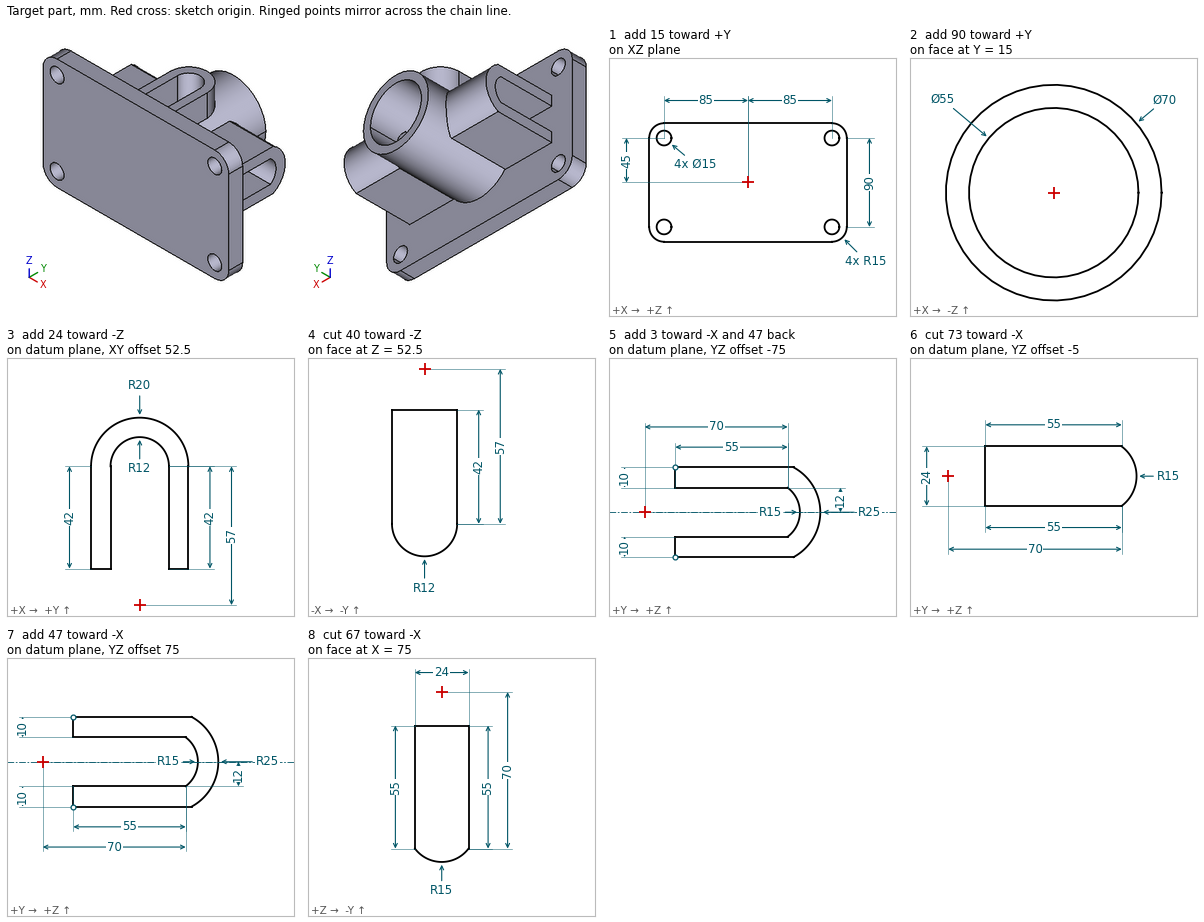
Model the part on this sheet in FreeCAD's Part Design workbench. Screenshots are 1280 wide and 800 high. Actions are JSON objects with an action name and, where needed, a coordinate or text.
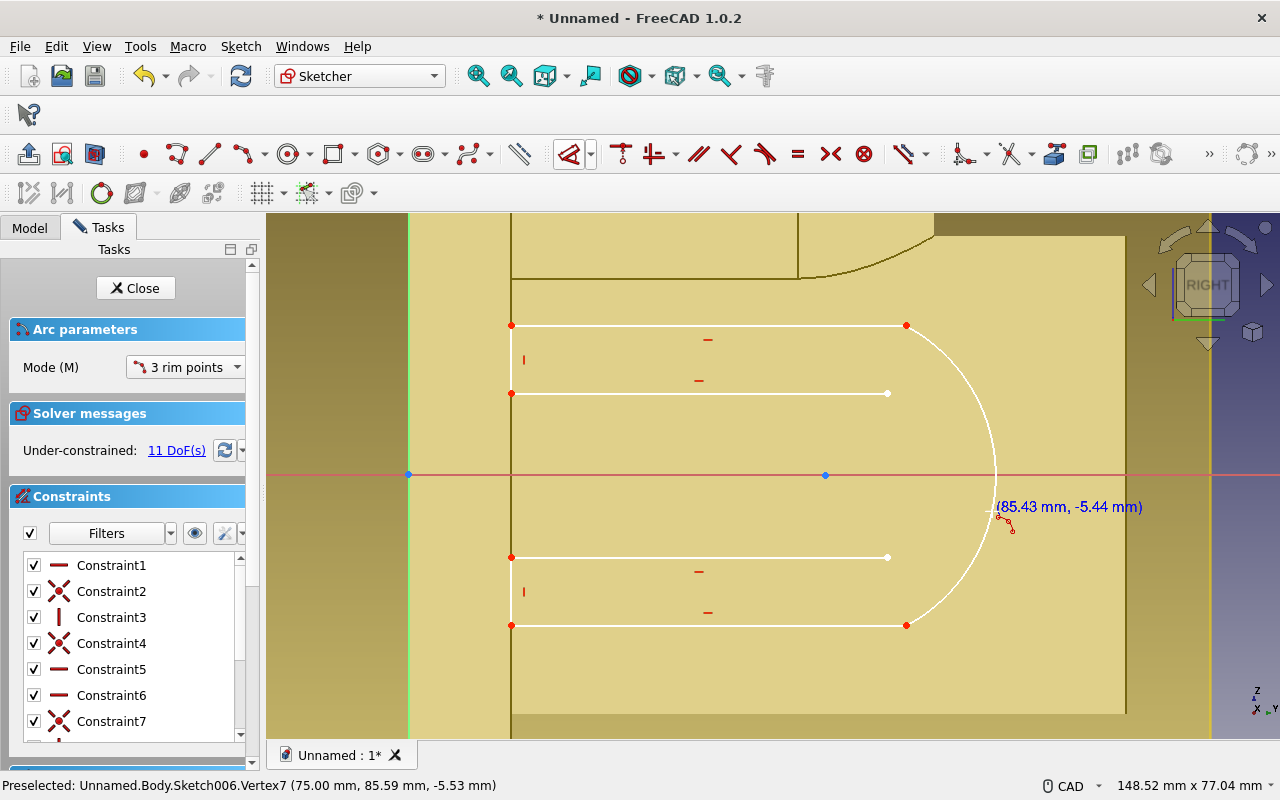
{"action": "left_click", "coordinate": [887, 394]}
{"action": "left_click", "coordinate": [887, 558]}
{"action": "left_click", "coordinate": [926, 494]}
{"action": "key", "text": "Escape"}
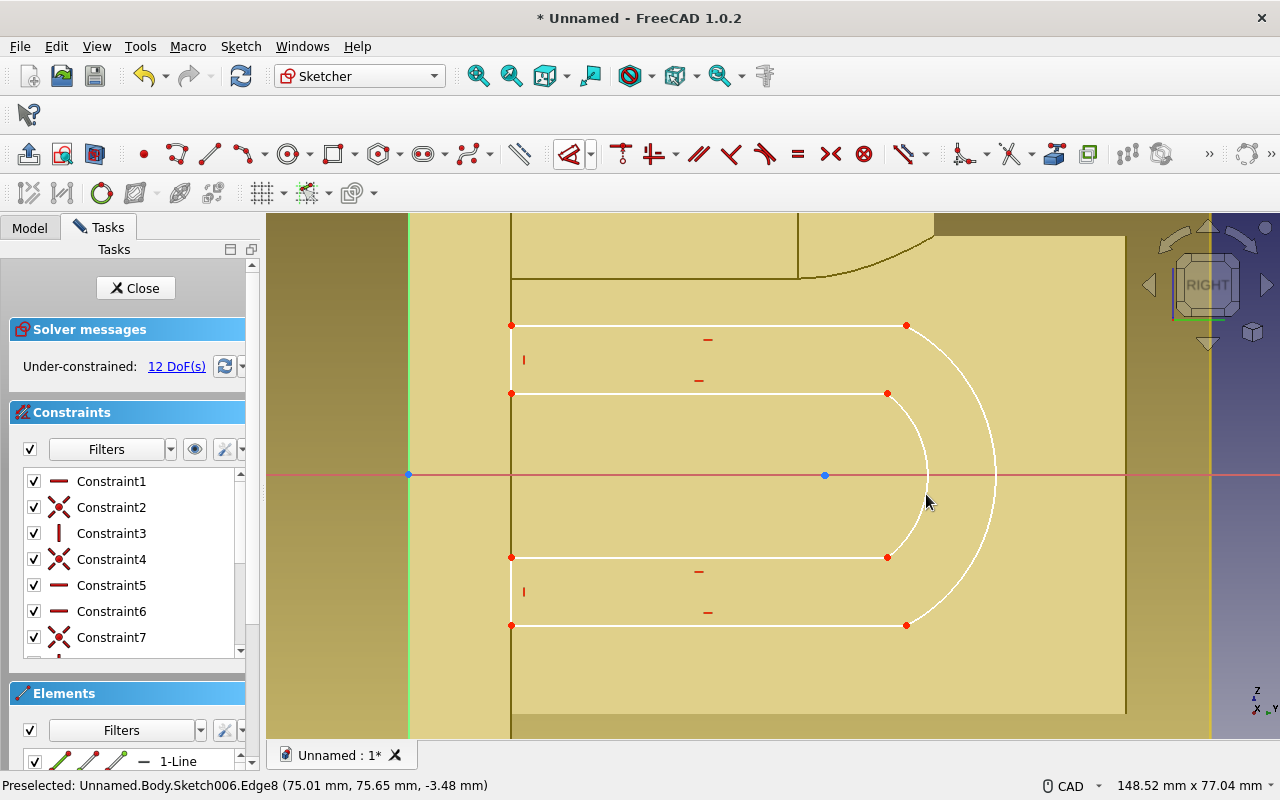
{"action": "left_click", "coordinate": [980, 547]}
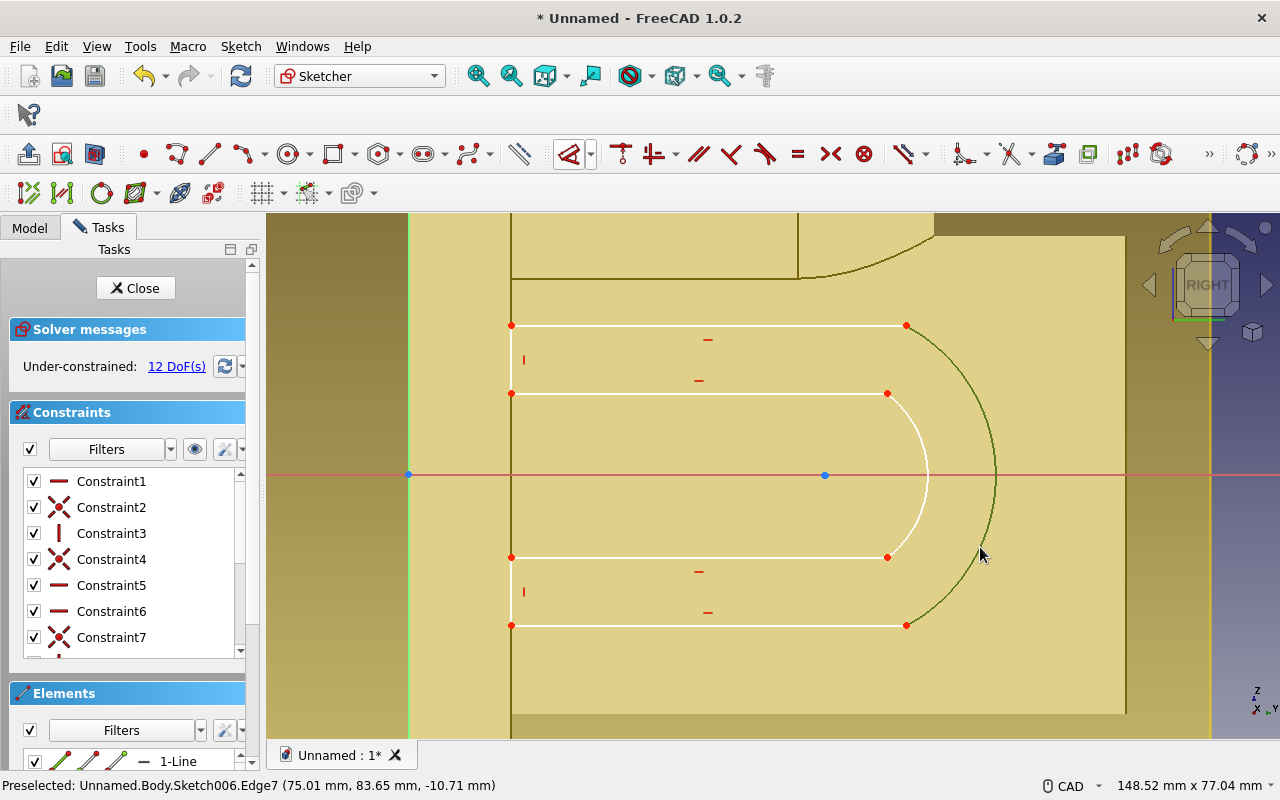
{"action": "left_click", "coordinate": [921, 513]}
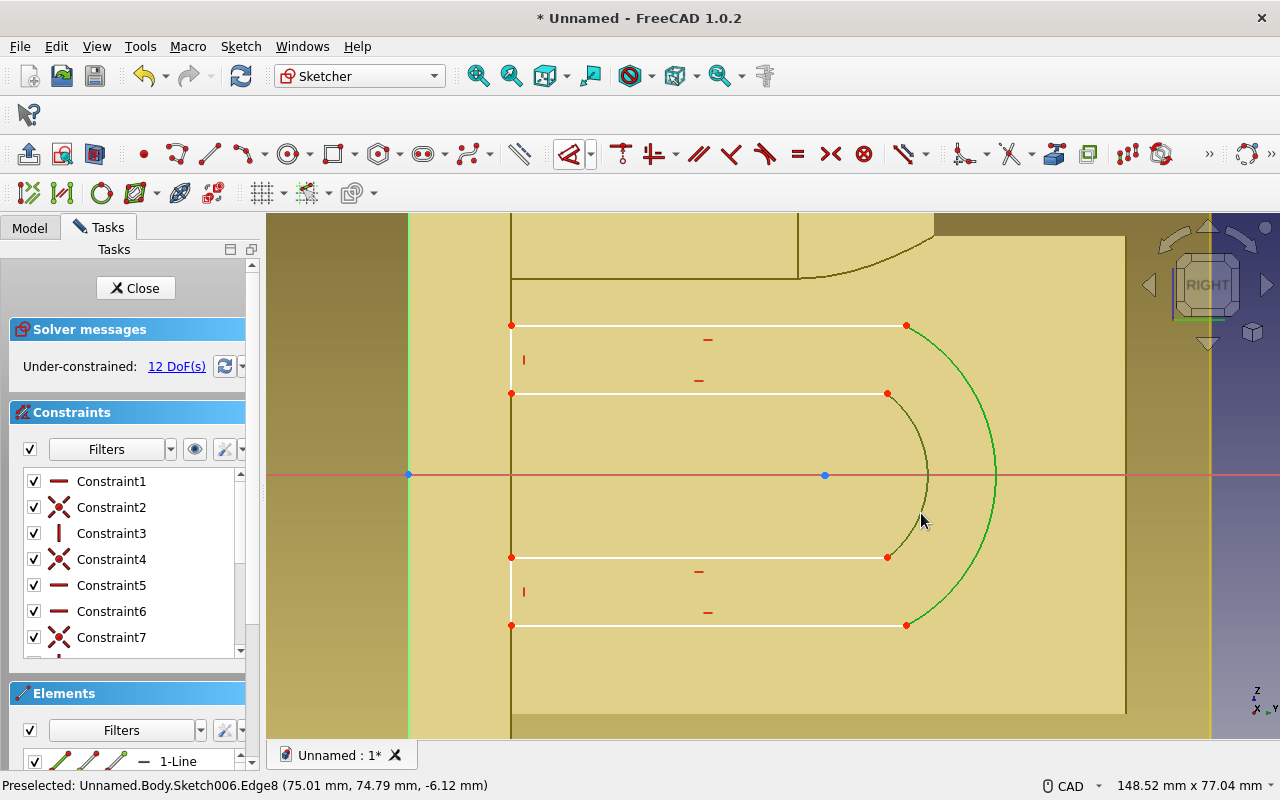
{"action": "key", "text": "c"}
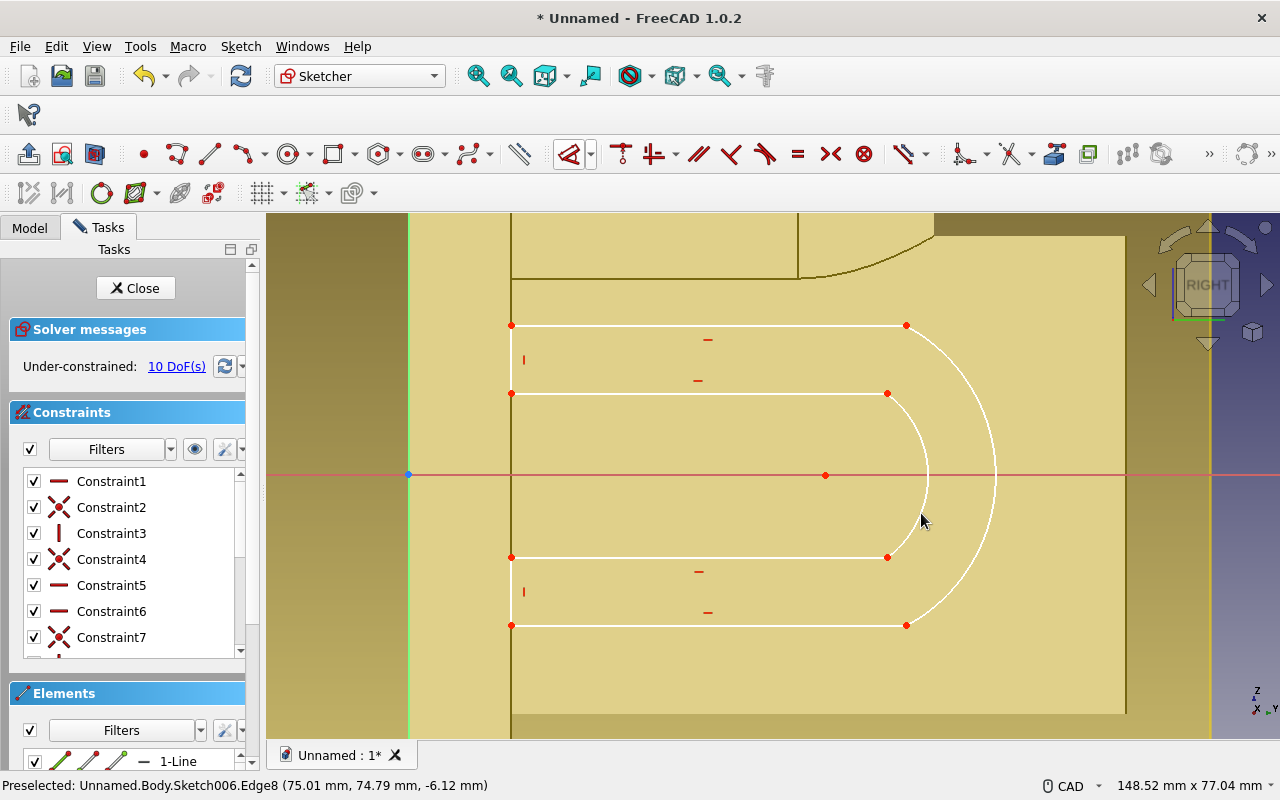
{"action": "left_click", "coordinate": [826, 476]}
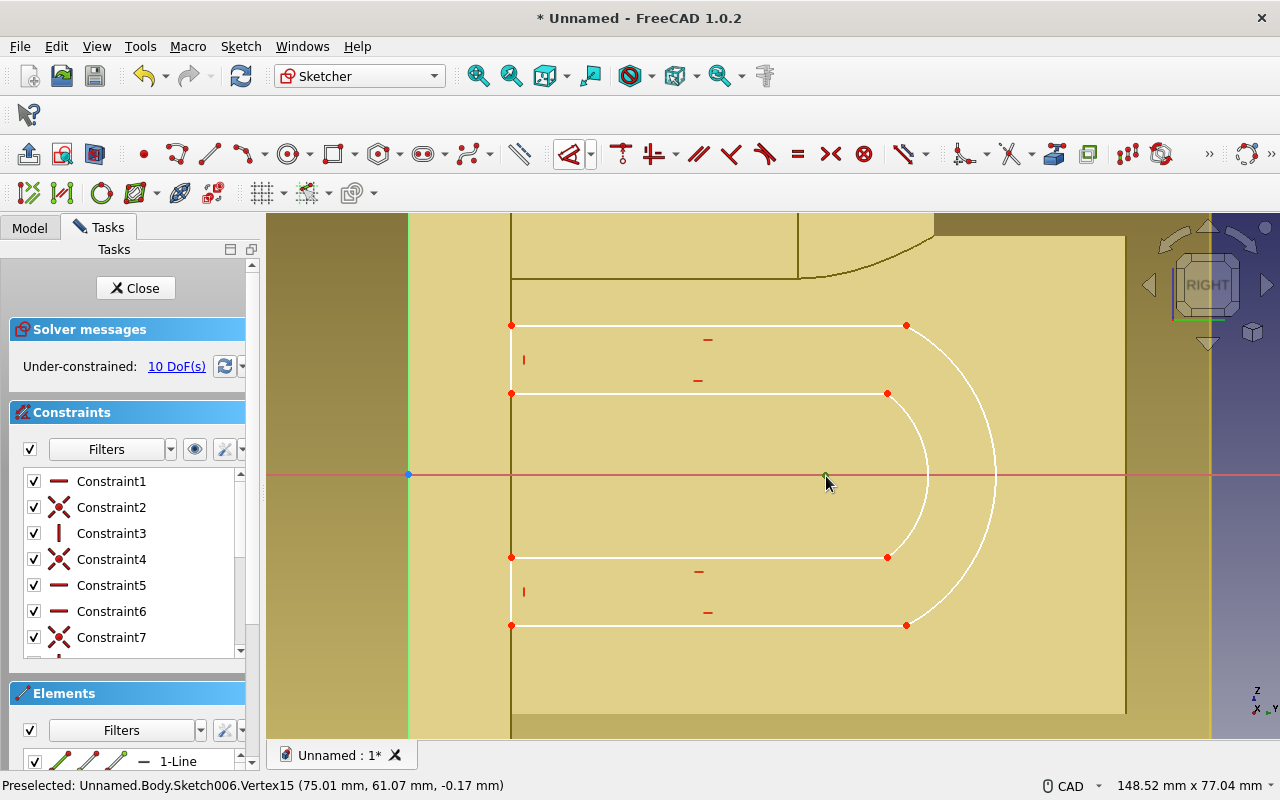
{"action": "left_click", "coordinate": [353, 475]}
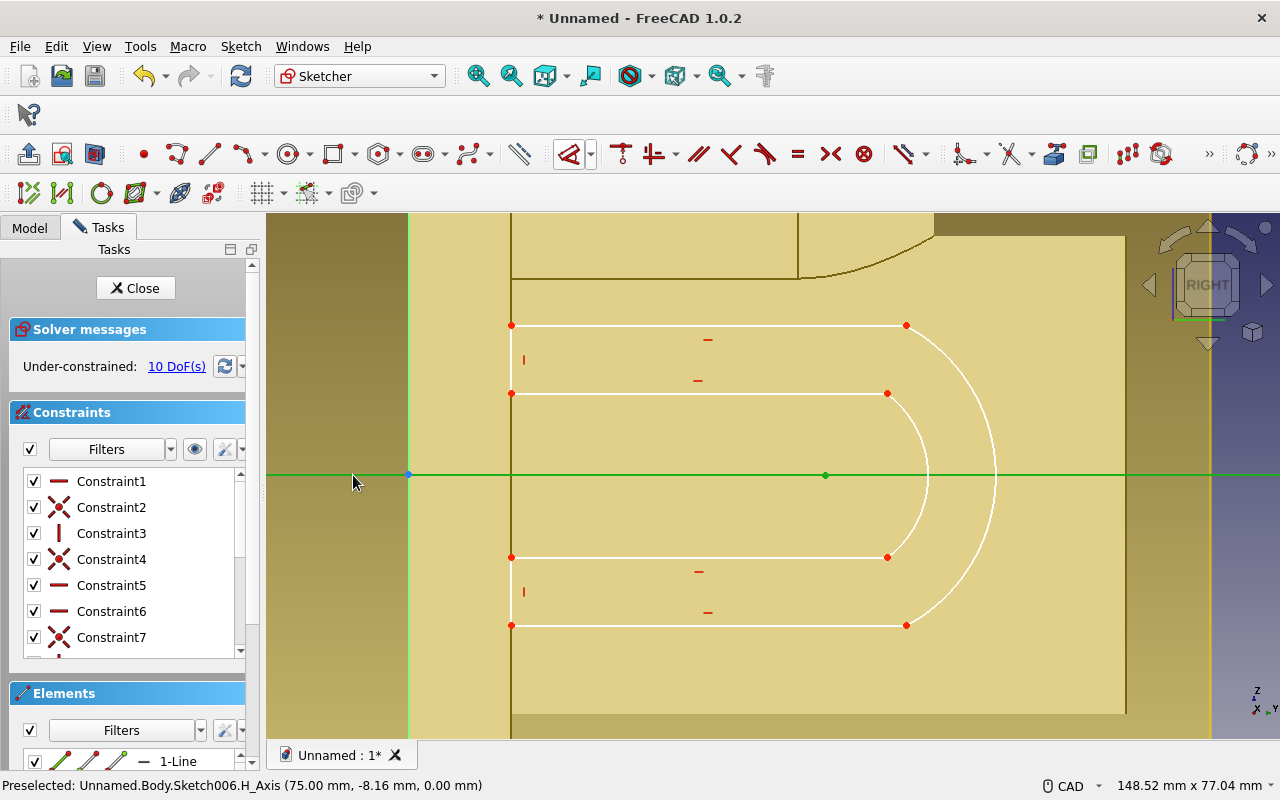
{"action": "key", "text": "c"}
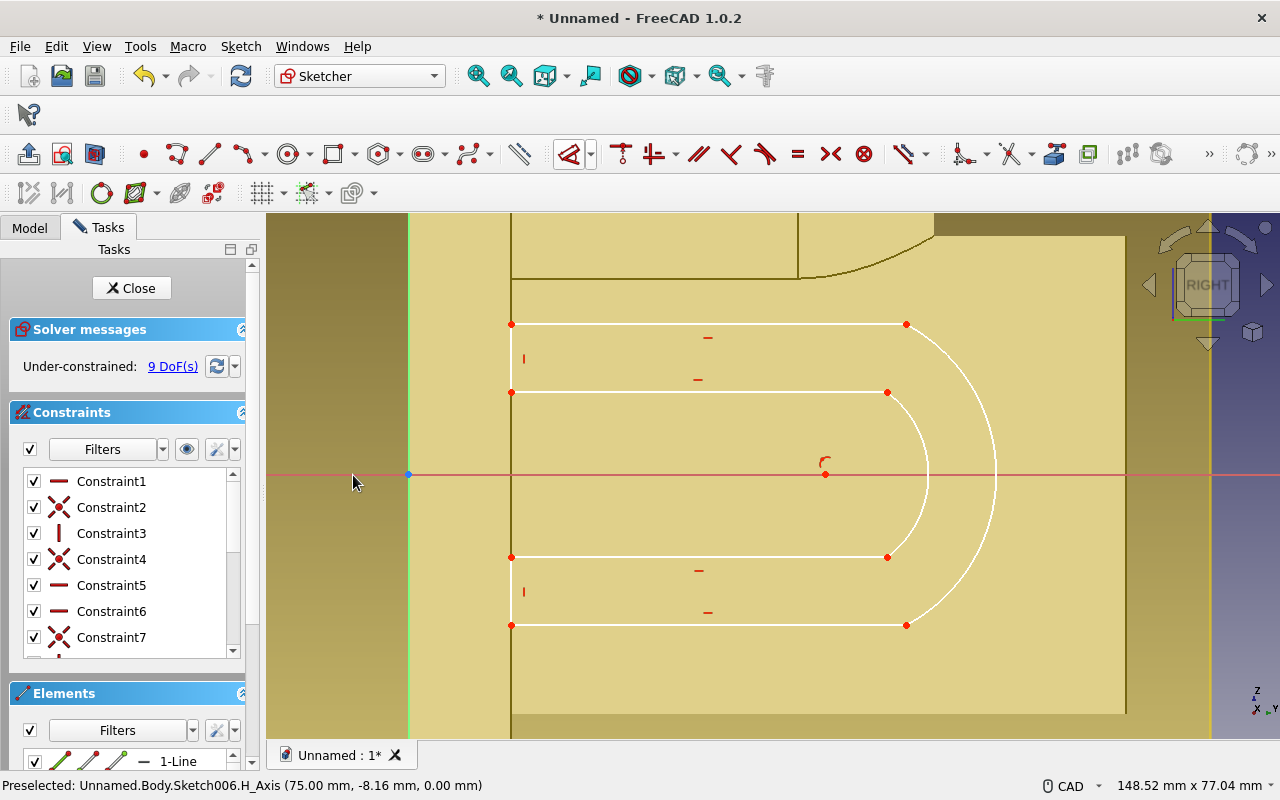
{"action": "left_click", "coordinate": [511, 625]}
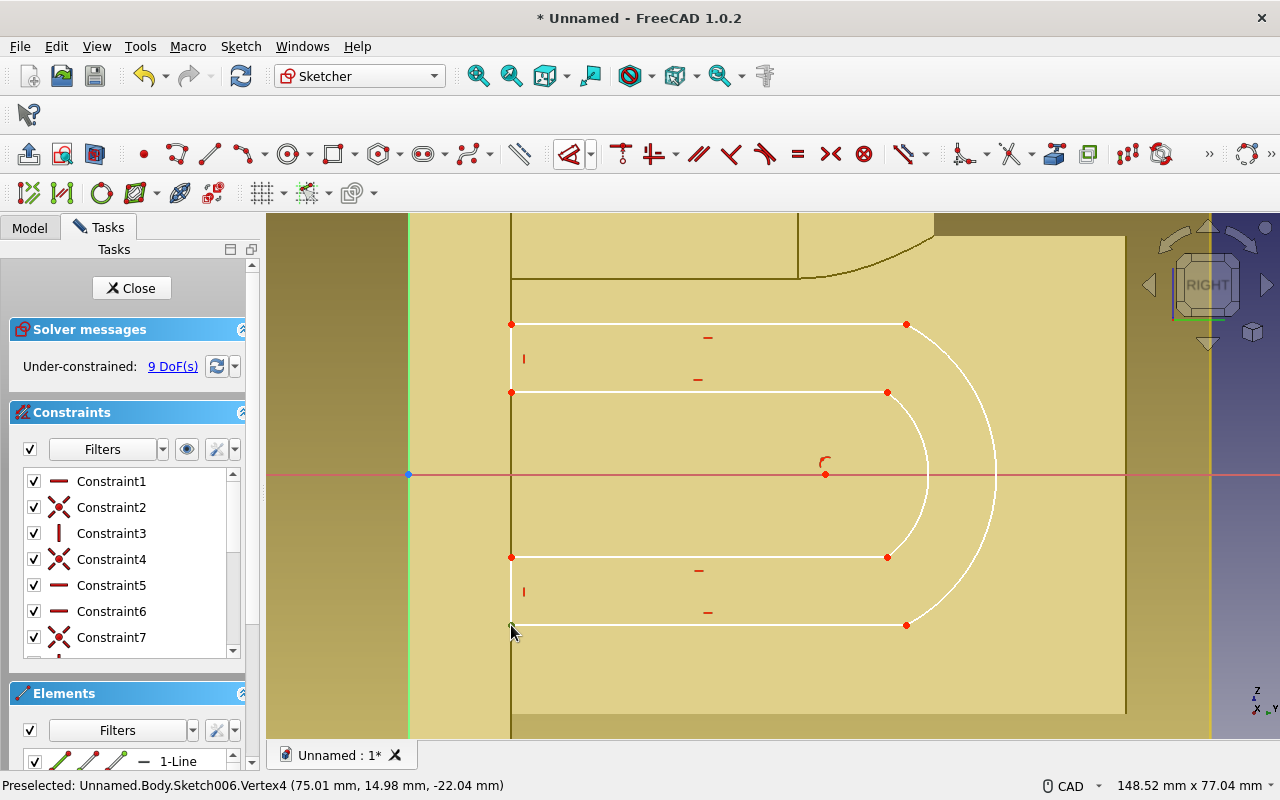
{"action": "left_click", "coordinate": [511, 324]}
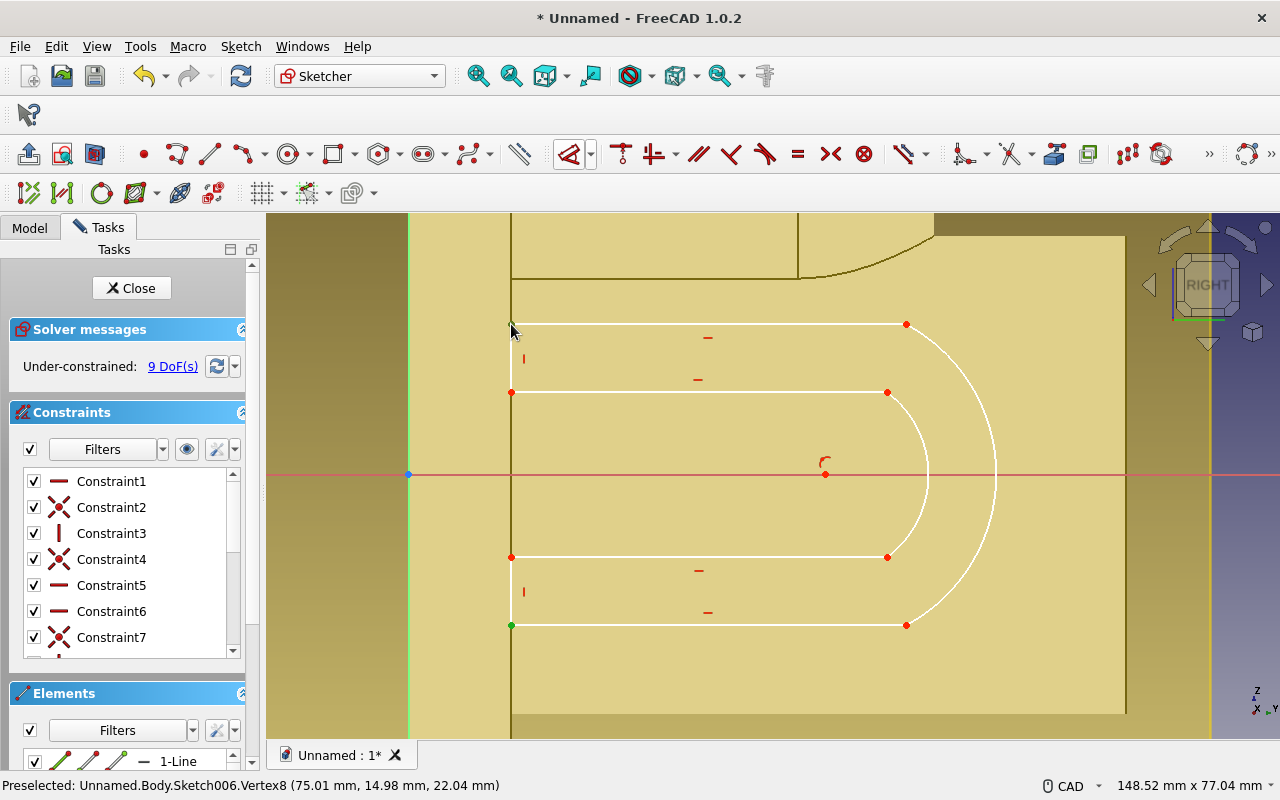
{"action": "left_click", "coordinate": [353, 475]}